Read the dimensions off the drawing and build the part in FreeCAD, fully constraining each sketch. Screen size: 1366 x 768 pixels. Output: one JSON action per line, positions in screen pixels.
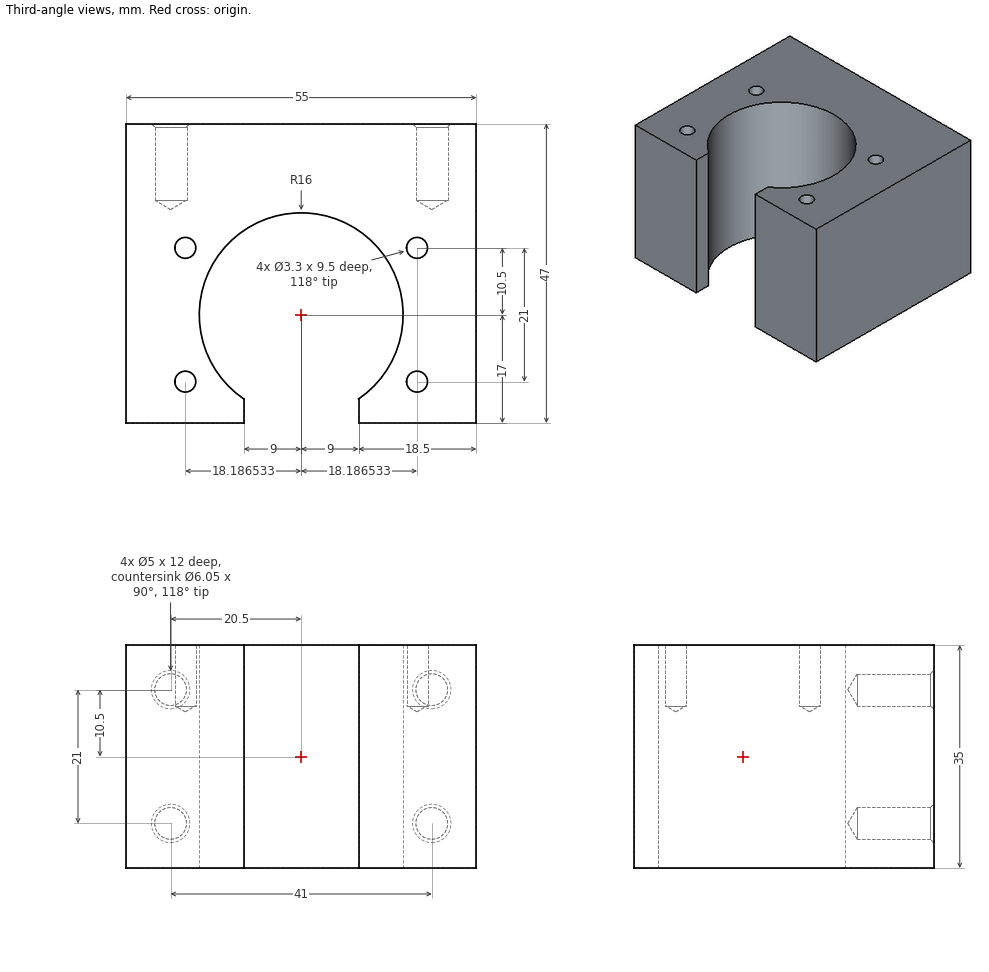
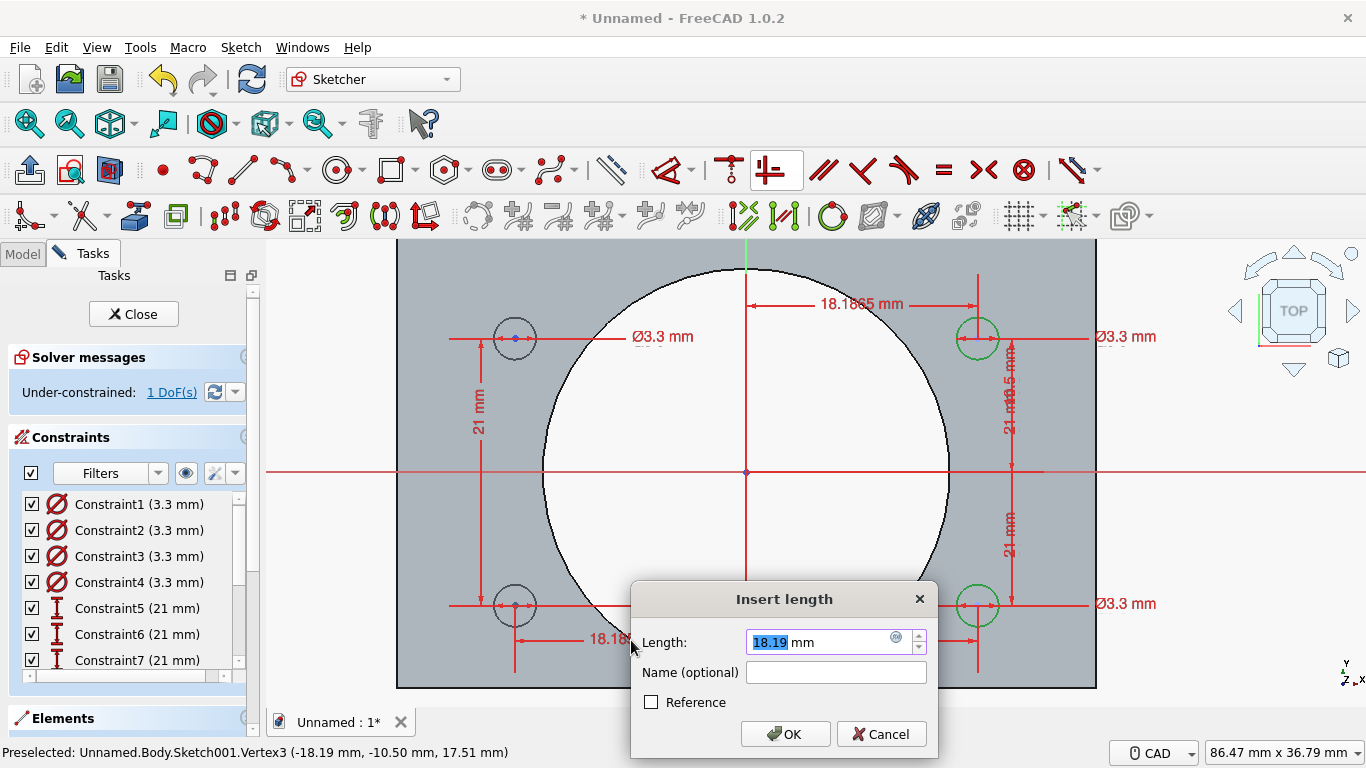
{"action": "type", "text": "18.186533"}
{"action": "key", "text": "Return"}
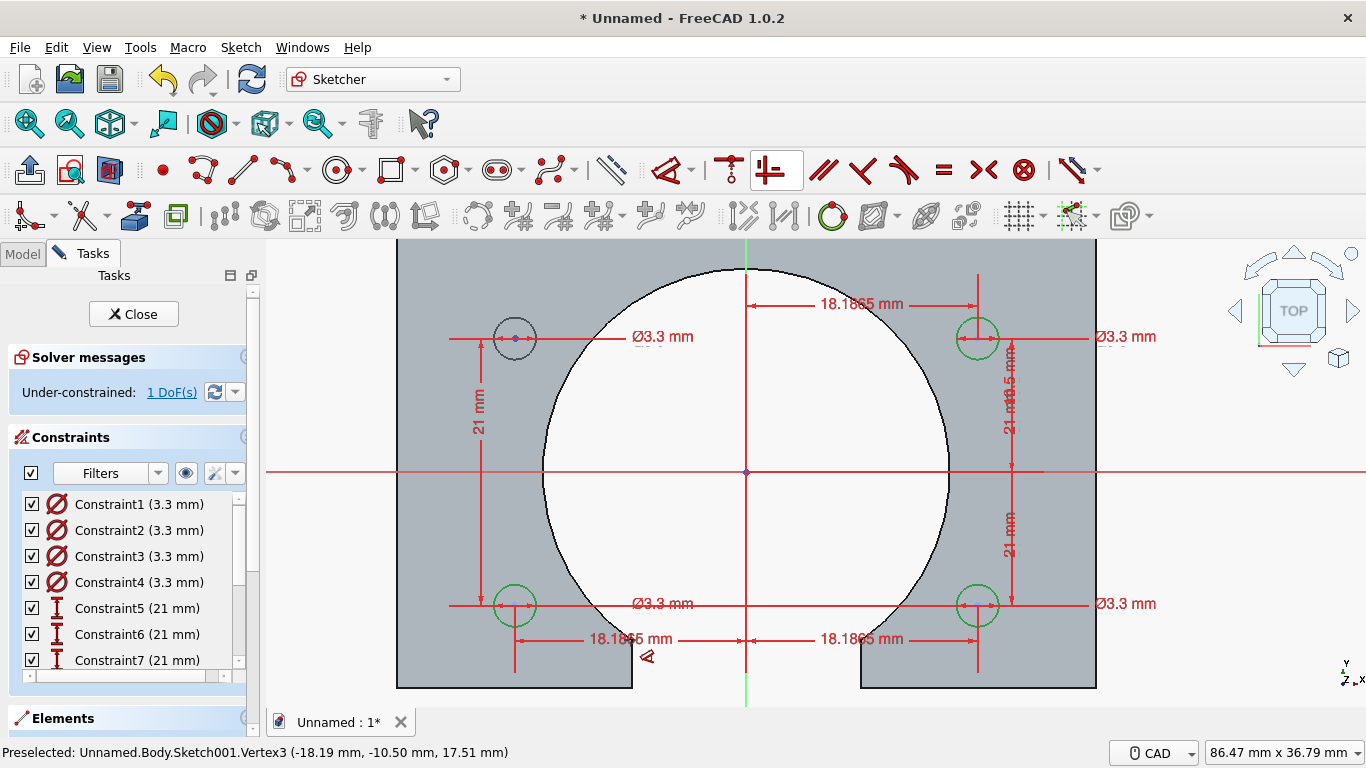
{"action": "left_click", "coordinate": [515, 339]}
{"action": "left_click", "coordinate": [631, 305]}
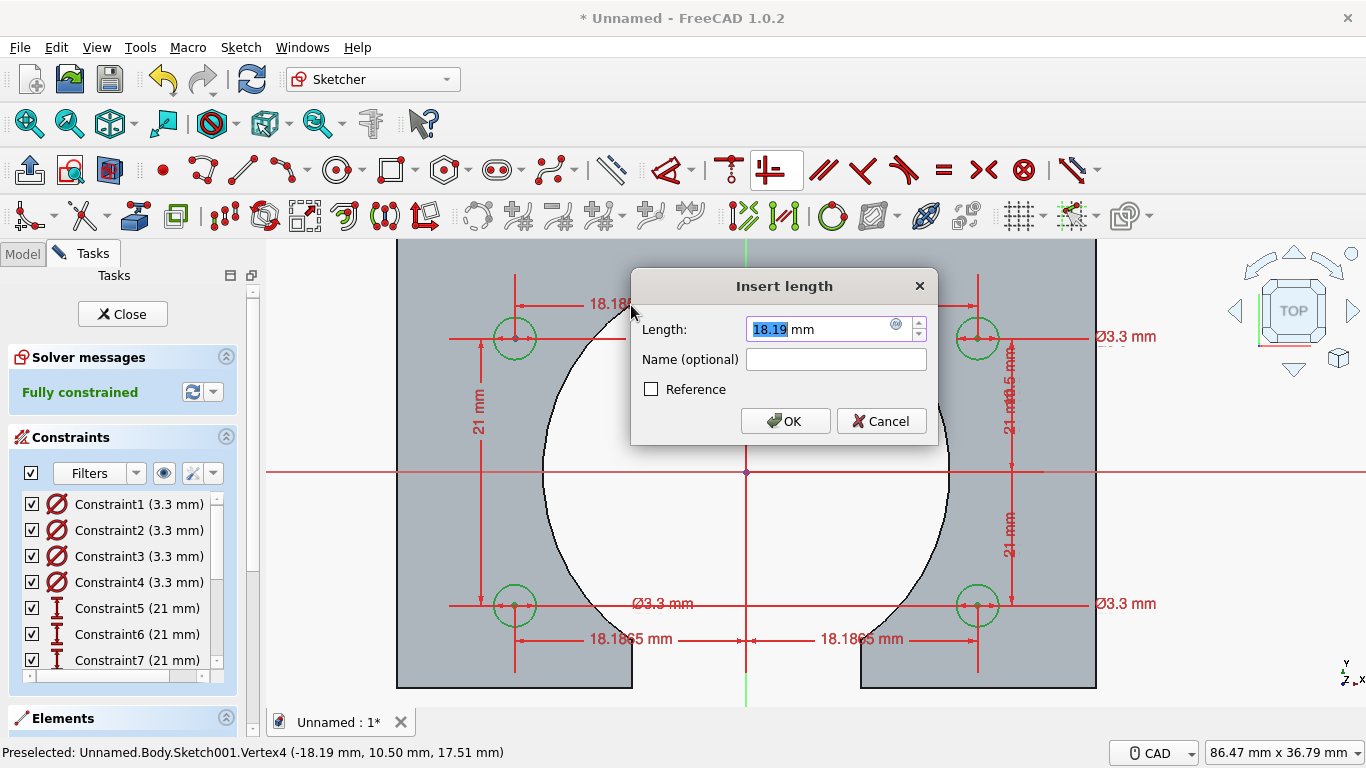
{"action": "type", "text": "18.186533"}
{"action": "key", "text": "Return"}
{"action": "key", "text": "Escape"}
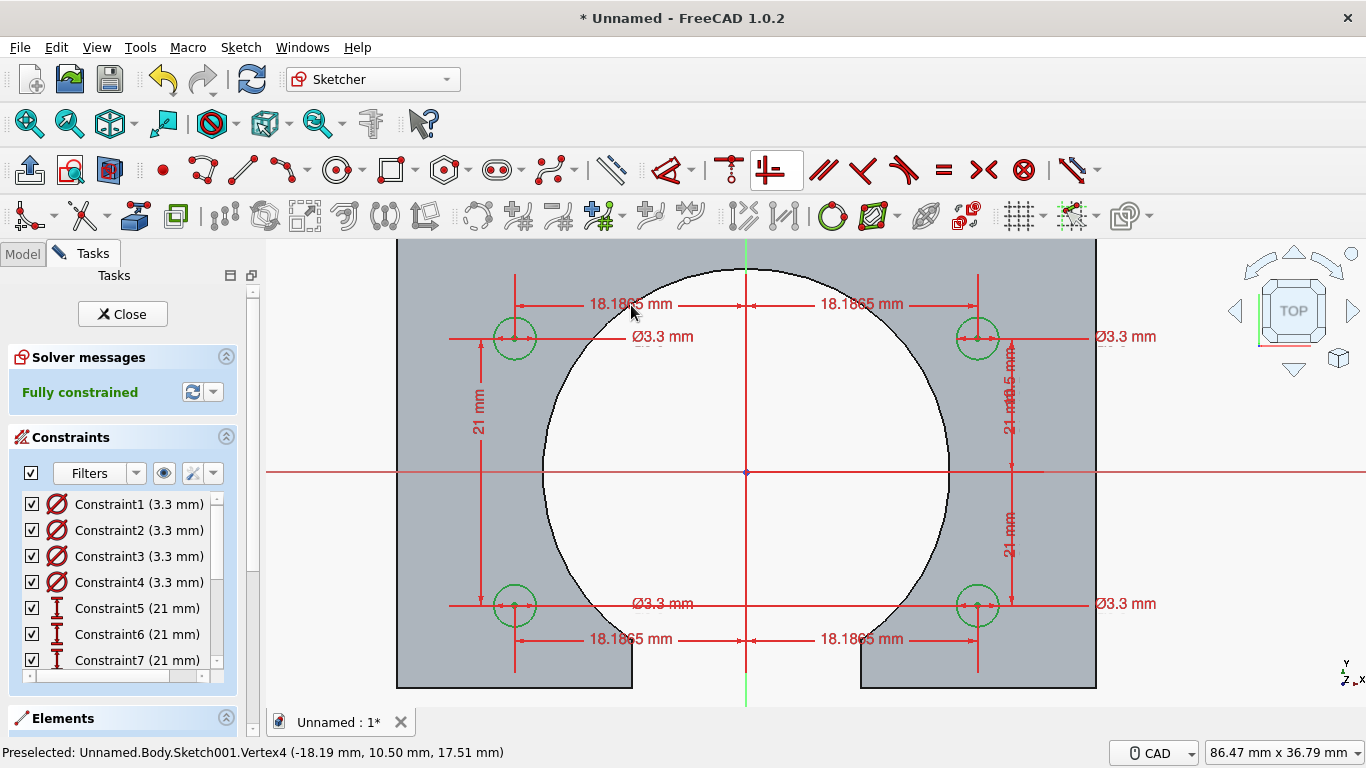
{"action": "left_click", "coordinate": [123, 314]}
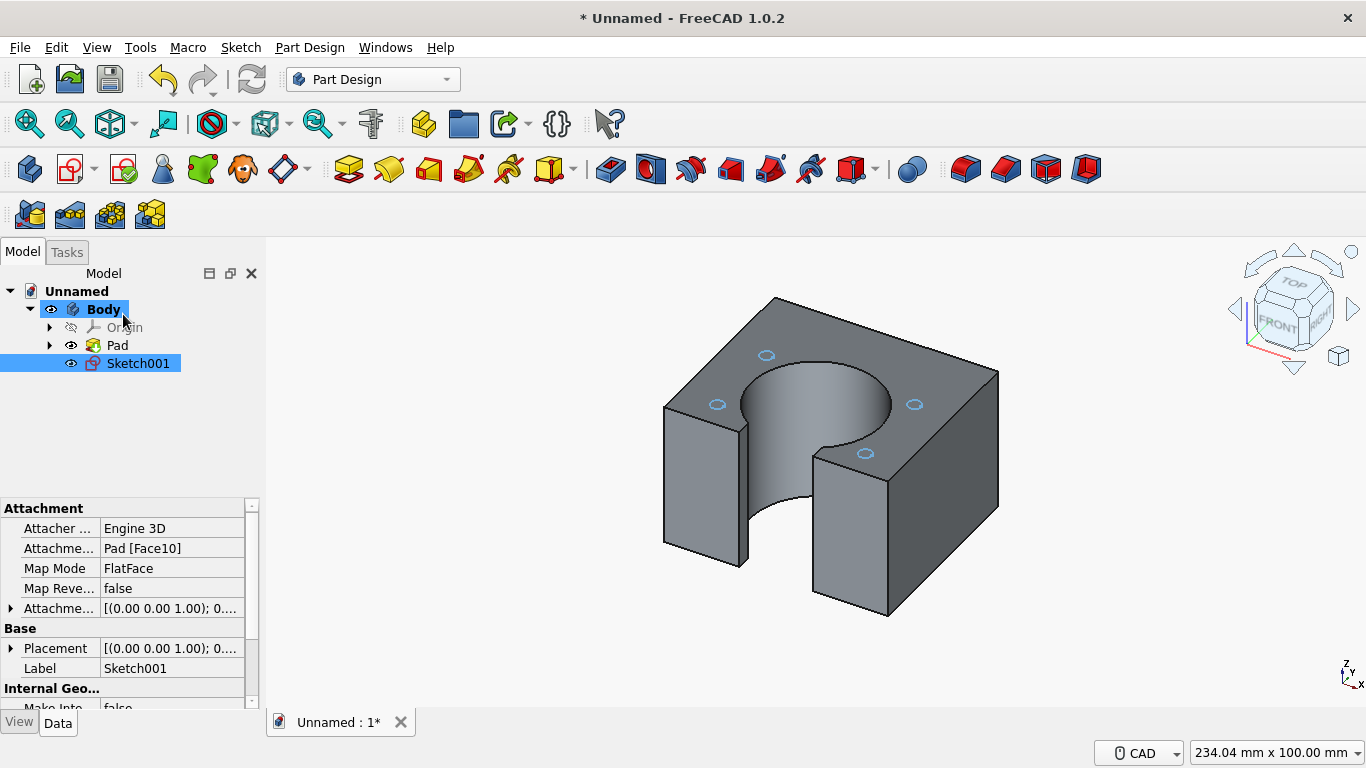
{"action": "left_click", "coordinate": [652, 170]}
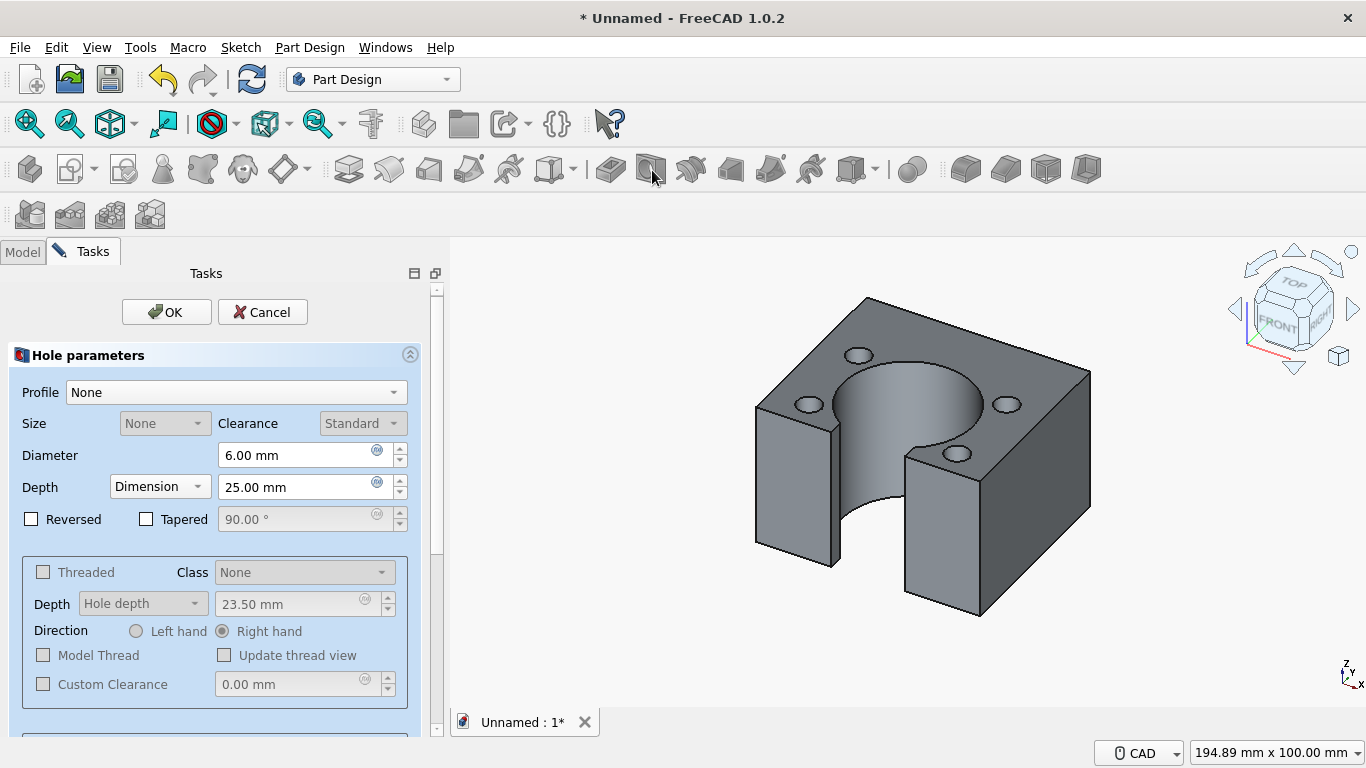
{"action": "triple_click", "coordinate": [305, 455]}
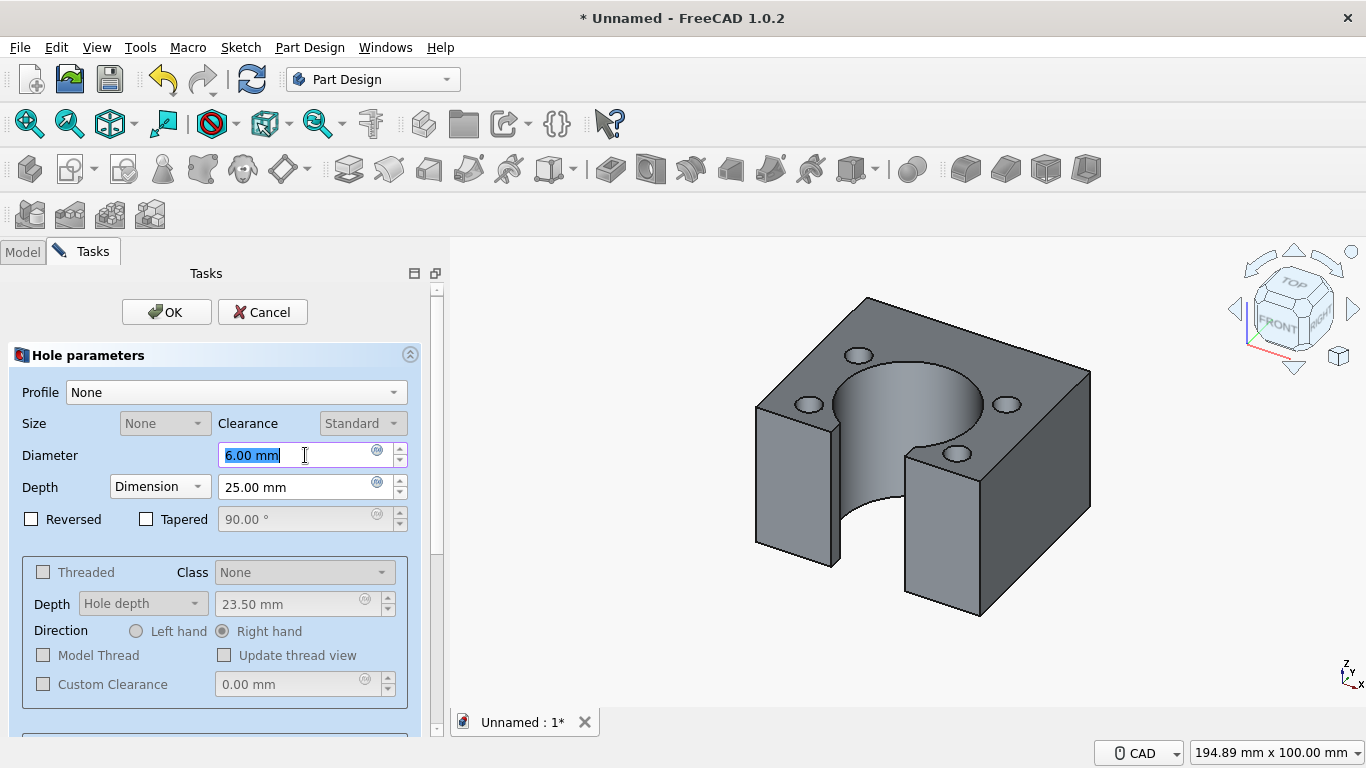
{"action": "type", "text": "3.3"}
{"action": "key", "text": "Tab"}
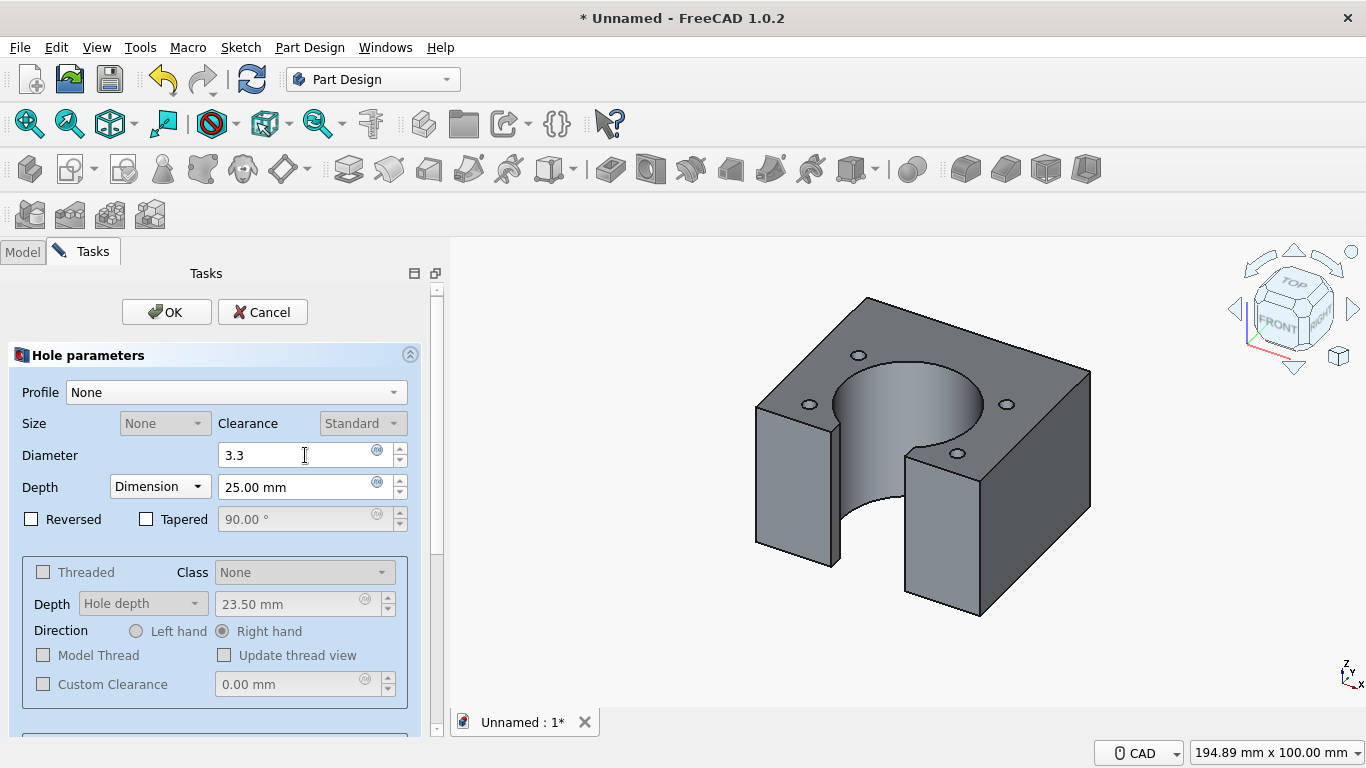
{"action": "triple_click", "coordinate": [305, 487]}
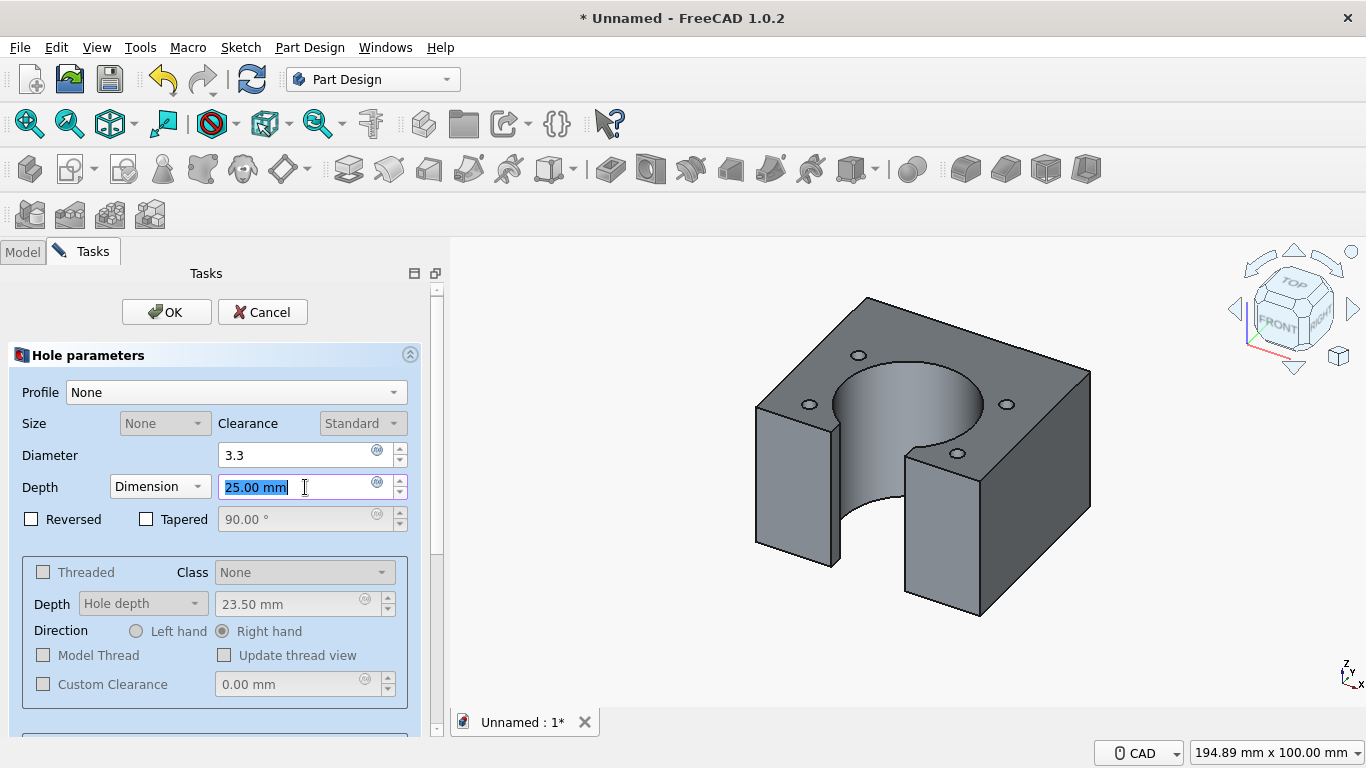
{"action": "type", "text": "9.5"}
{"action": "key", "text": "Tab"}